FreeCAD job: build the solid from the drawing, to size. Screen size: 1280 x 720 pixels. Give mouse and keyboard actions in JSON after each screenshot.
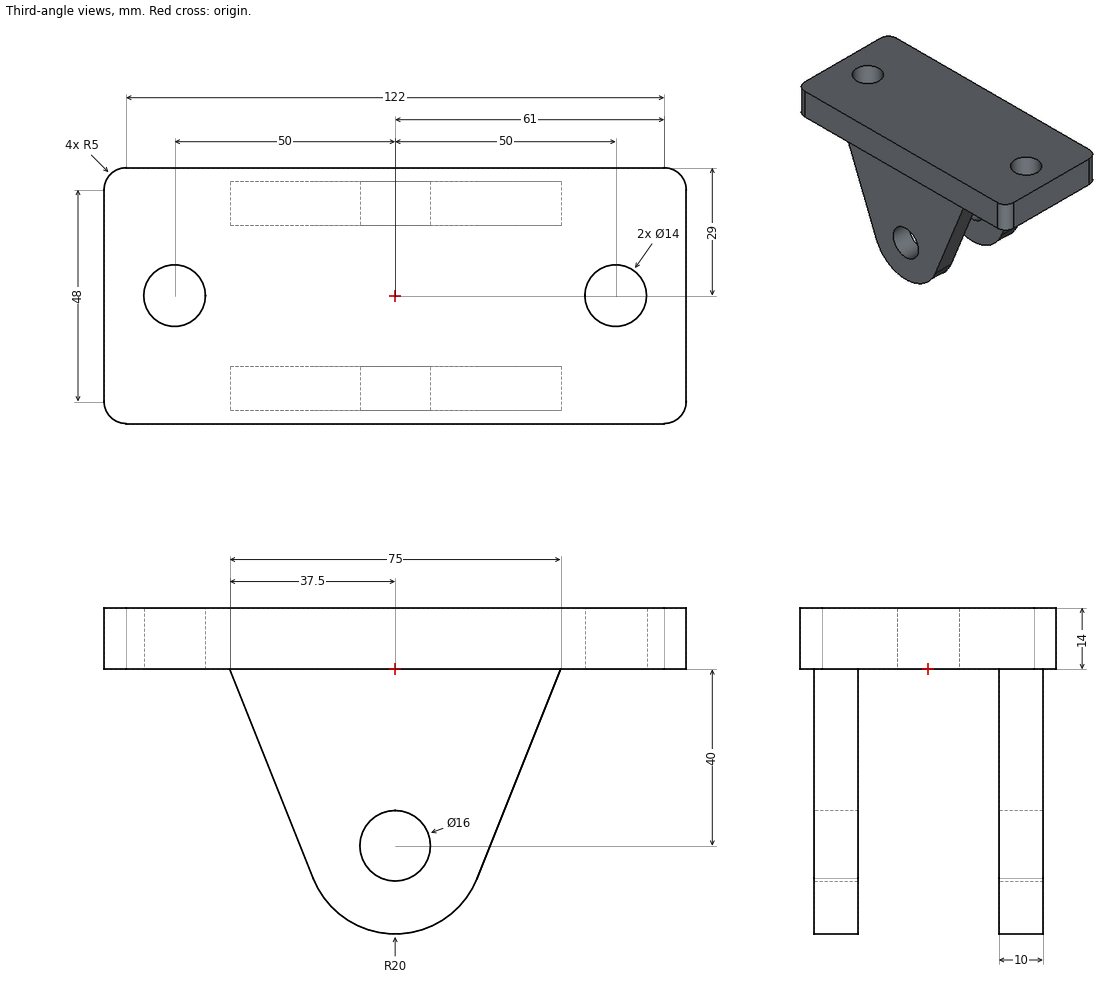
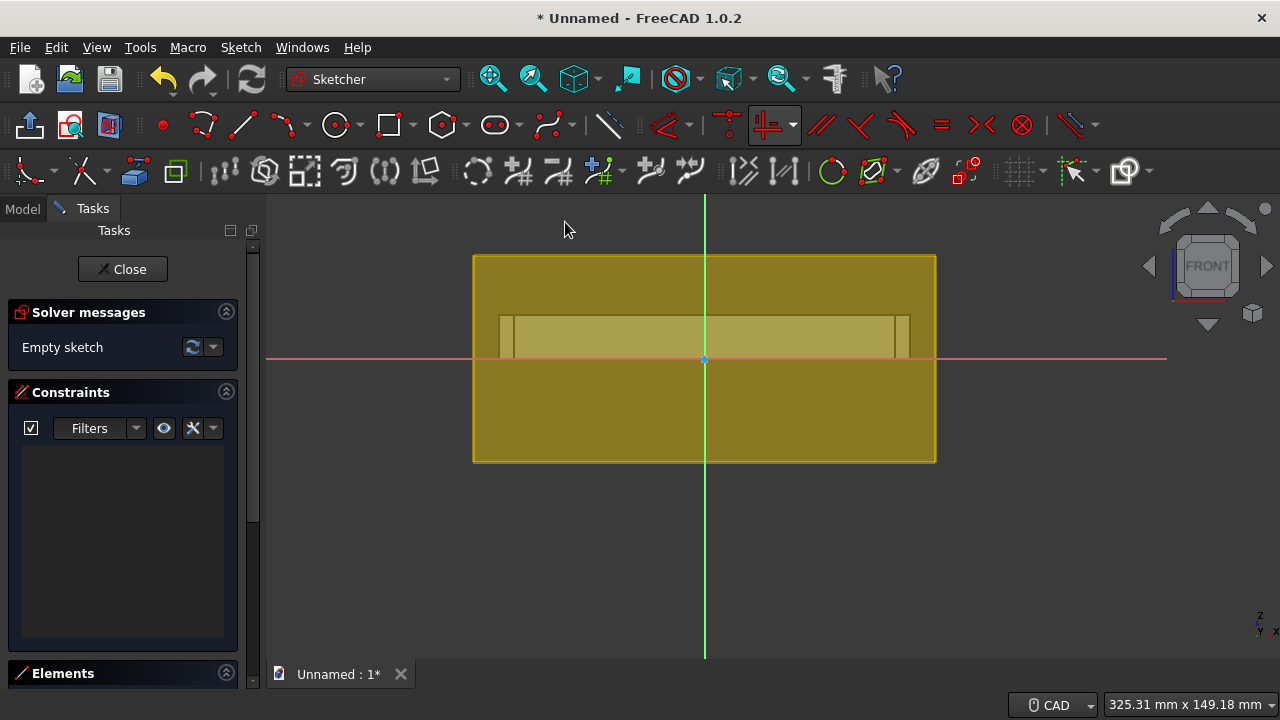
{"action": "scroll", "coordinate": [705, 506], "scroll_direction": "up", "scroll_amount": 2}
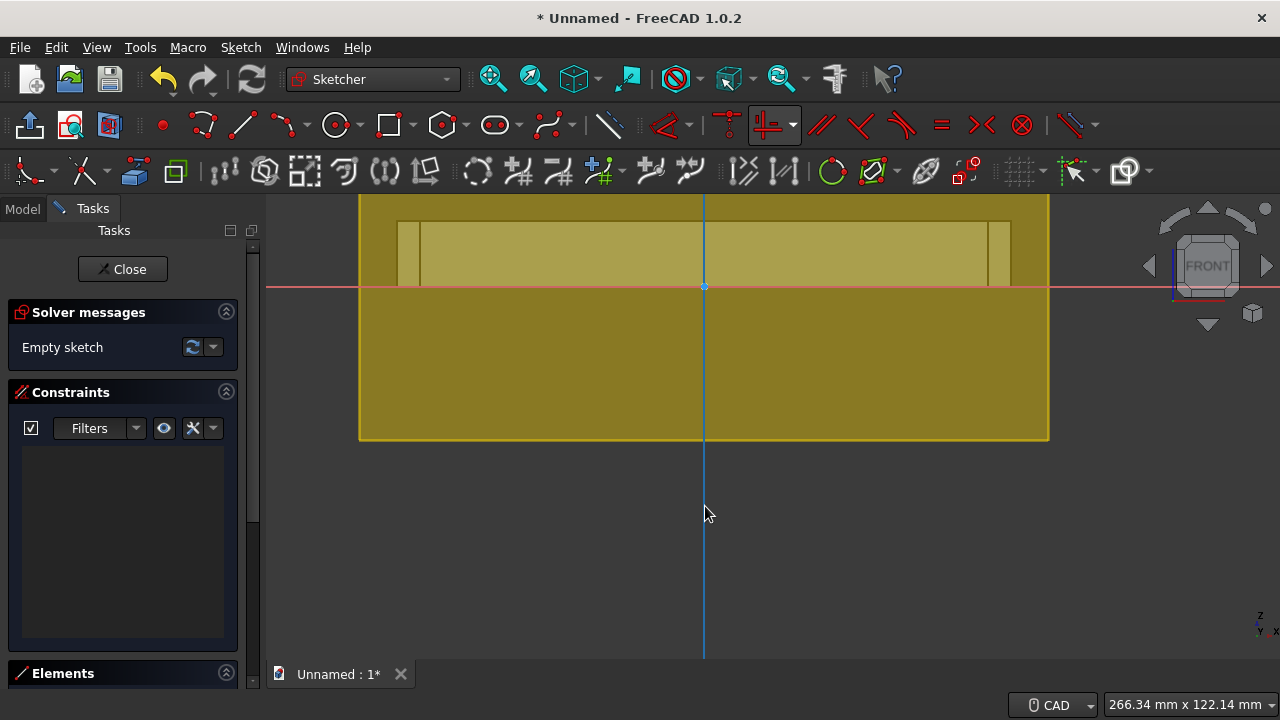
{"action": "left_click", "coordinate": [204, 126]}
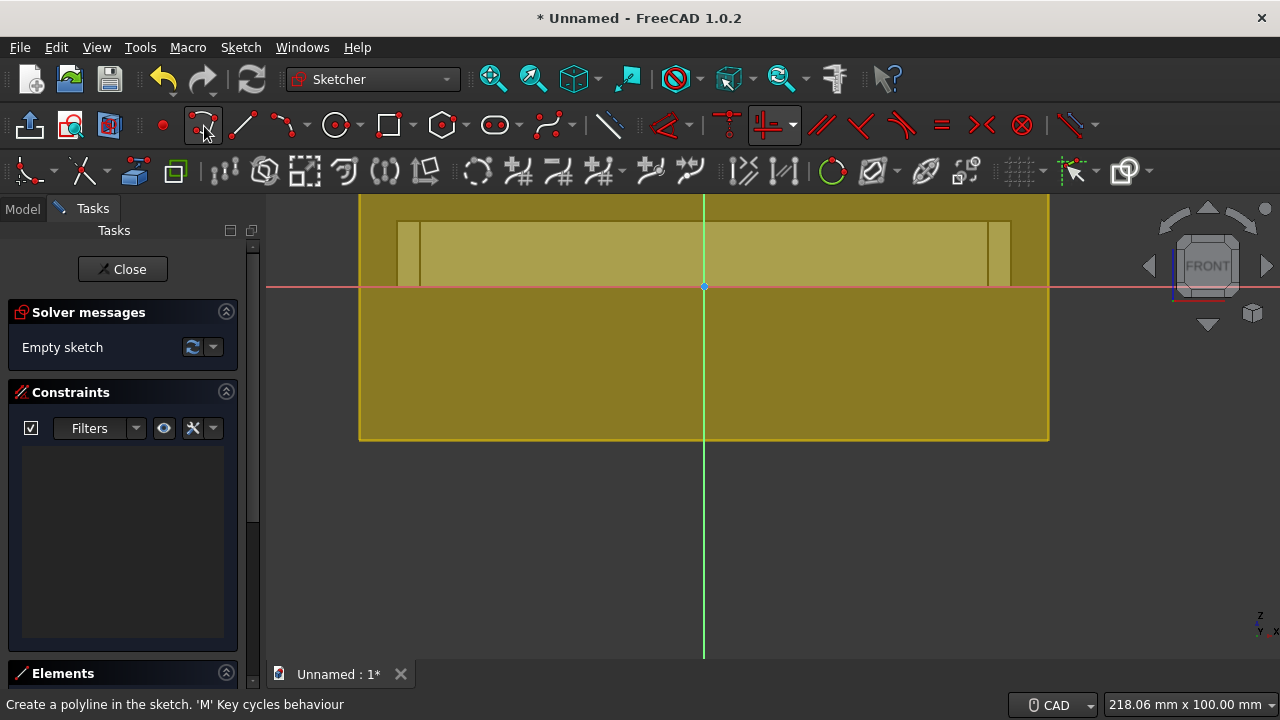
{"action": "left_click", "coordinate": [618, 507]}
{"action": "left_click", "coordinate": [530, 287]}
{"action": "left_click", "coordinate": [878, 296]}
{"action": "left_click", "coordinate": [790, 507]}
{"action": "right_click", "coordinate": [790, 507]}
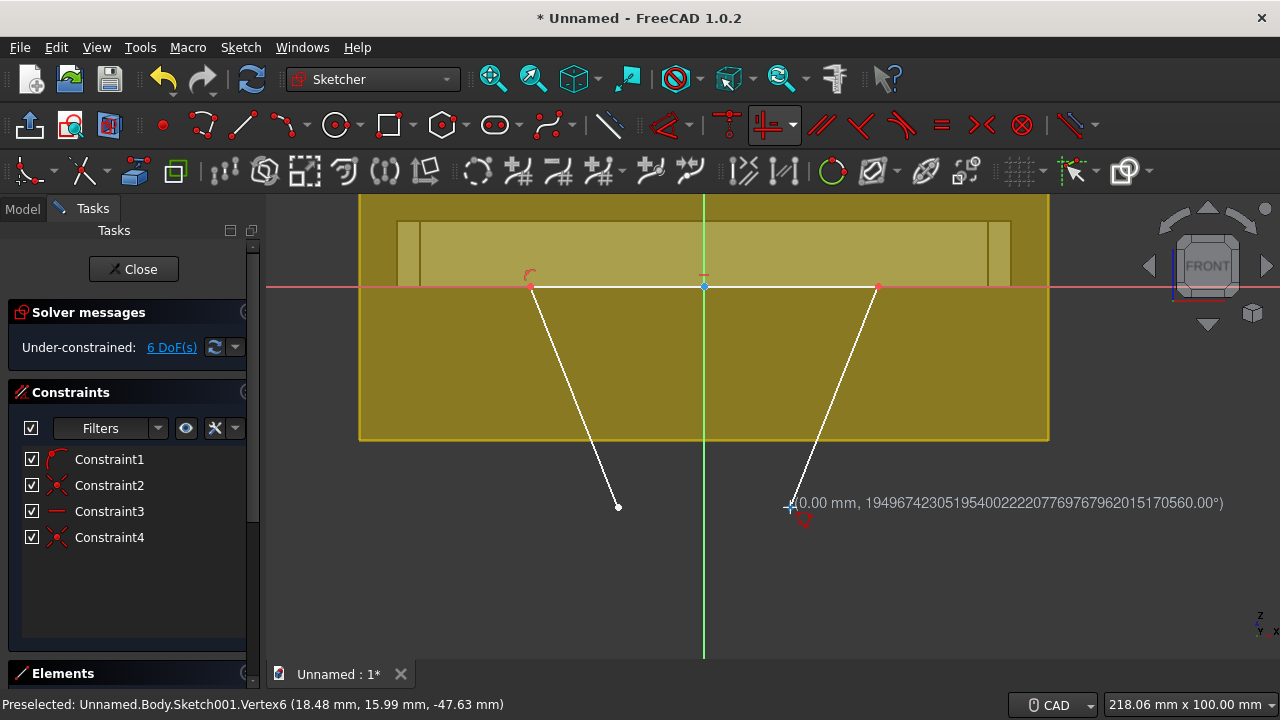
{"action": "left_click", "coordinate": [284, 126]}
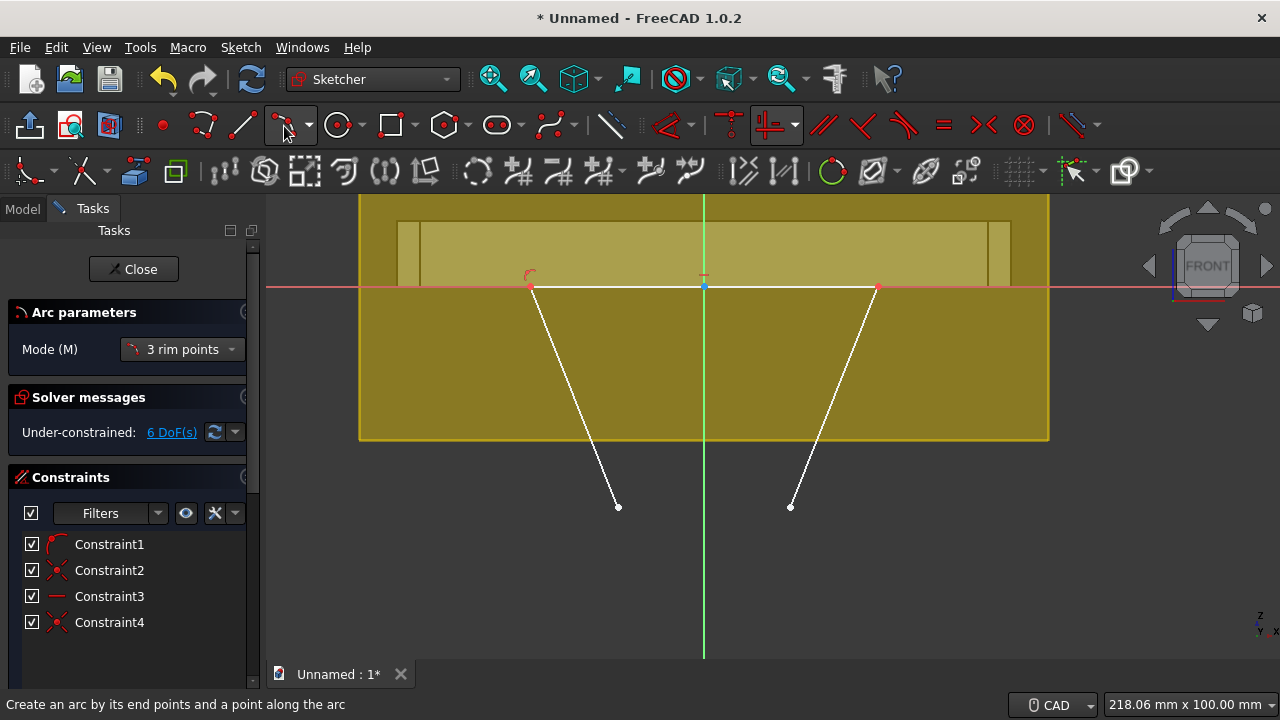
{"action": "left_click", "coordinate": [790, 508]}
{"action": "left_click", "coordinate": [618, 508]}
{"action": "left_click", "coordinate": [682, 563]}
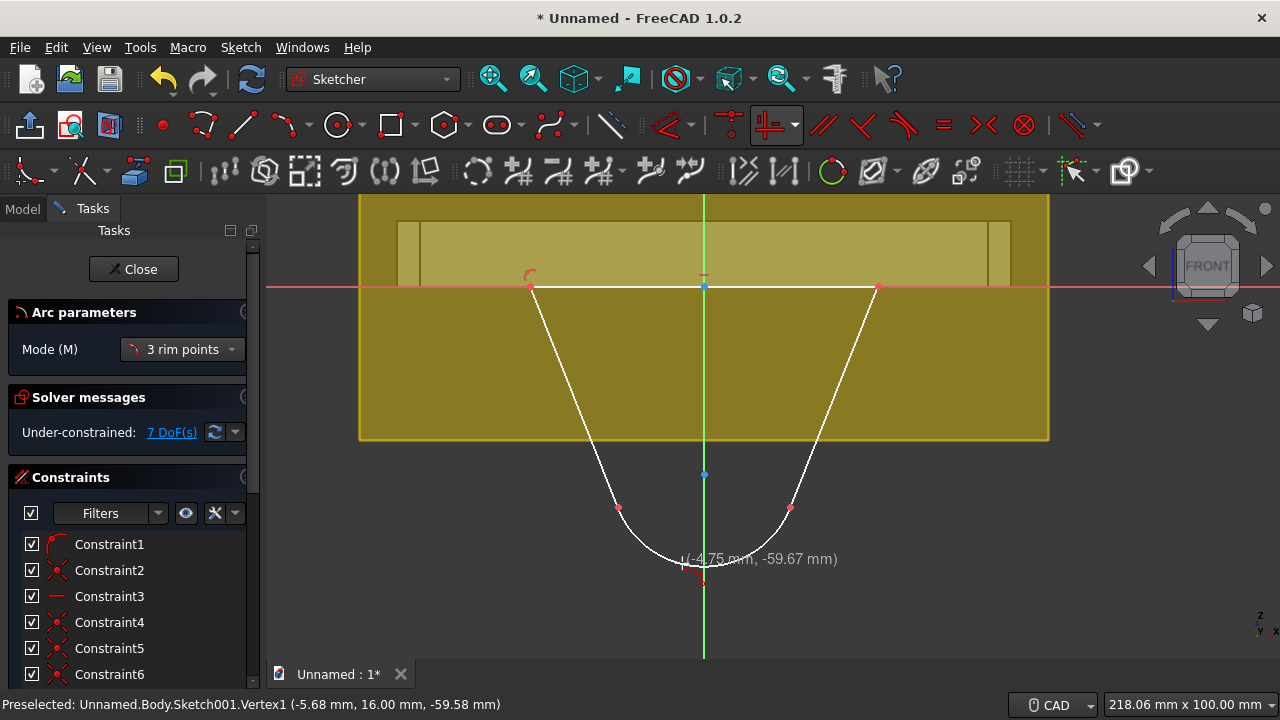
{"action": "left_click", "coordinate": [338, 126]}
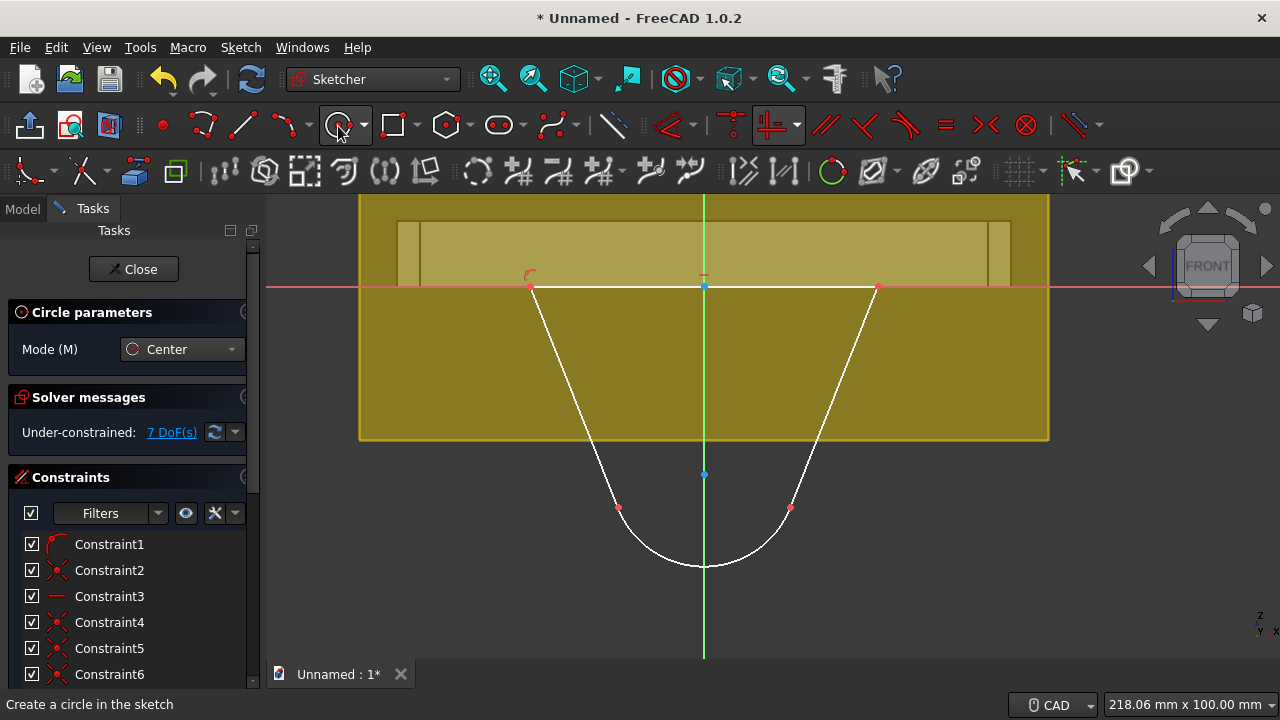
{"action": "left_click", "coordinate": [704, 473]}
{"action": "mouse_move", "coordinate": [730, 446]}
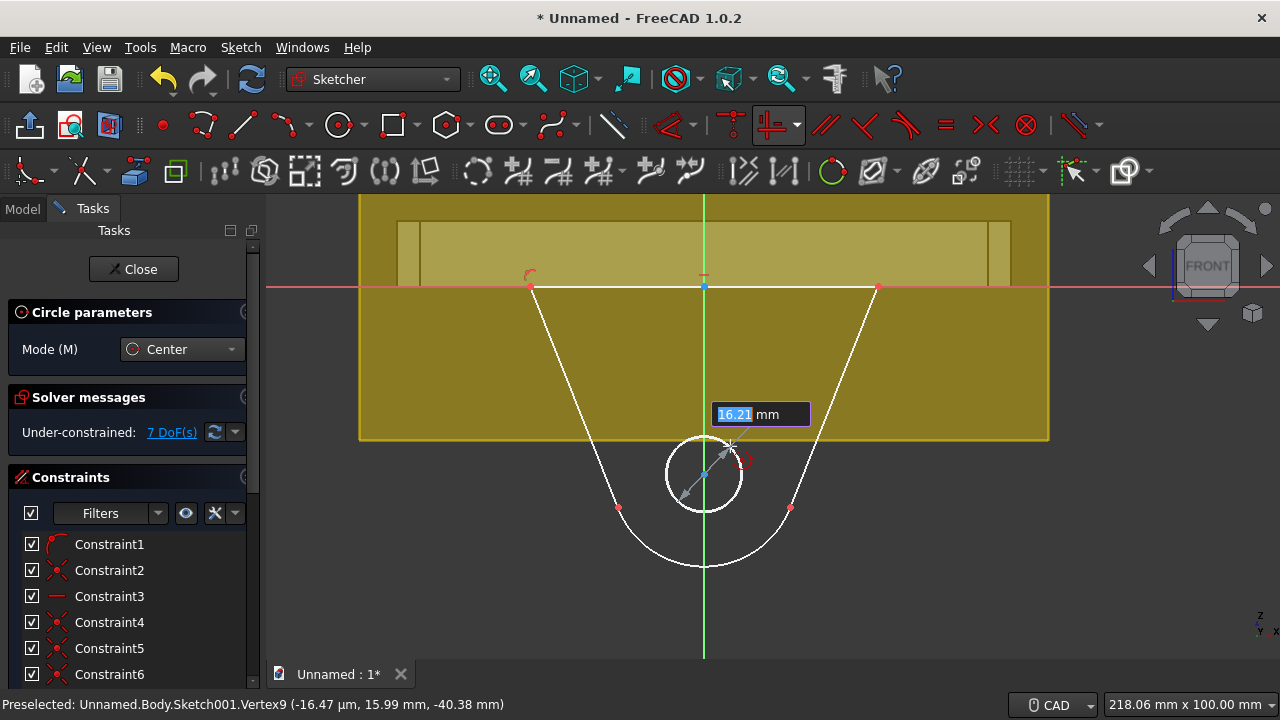
{"action": "type", "text": "16"}
{"action": "key", "text": "Return"}
{"action": "key", "text": "Escape"}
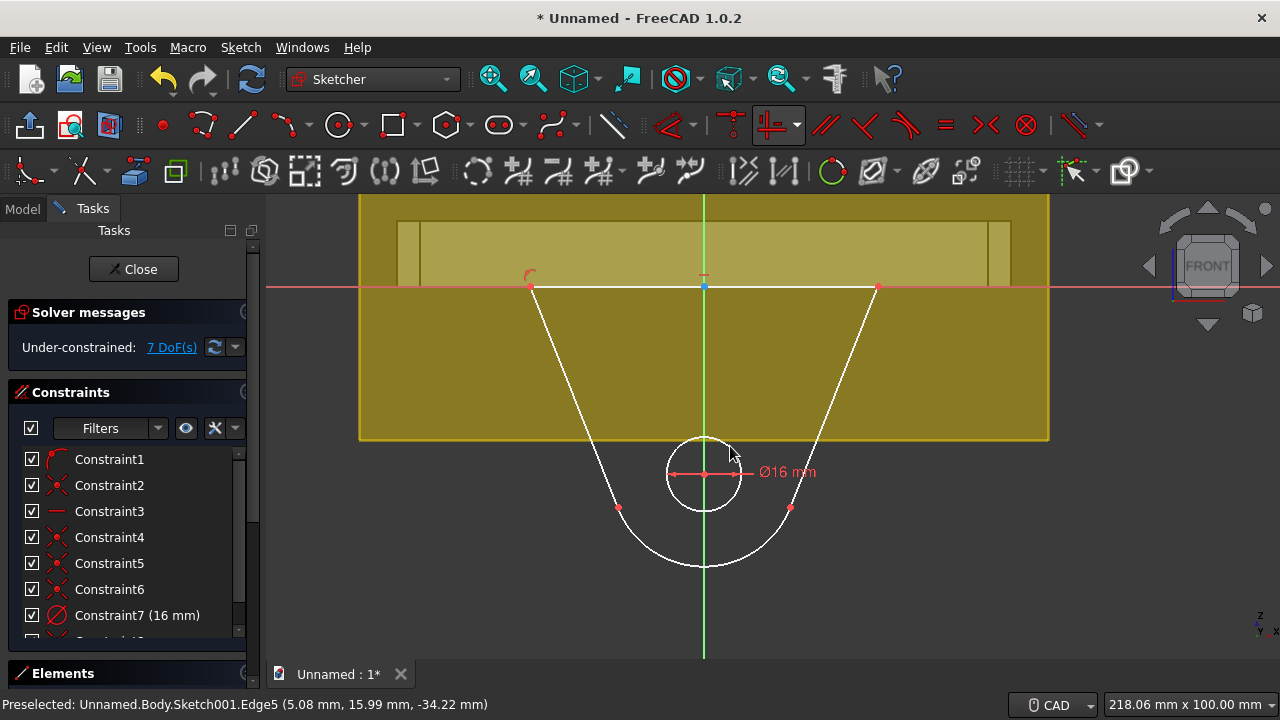
{"action": "left_click", "coordinate": [592, 442]}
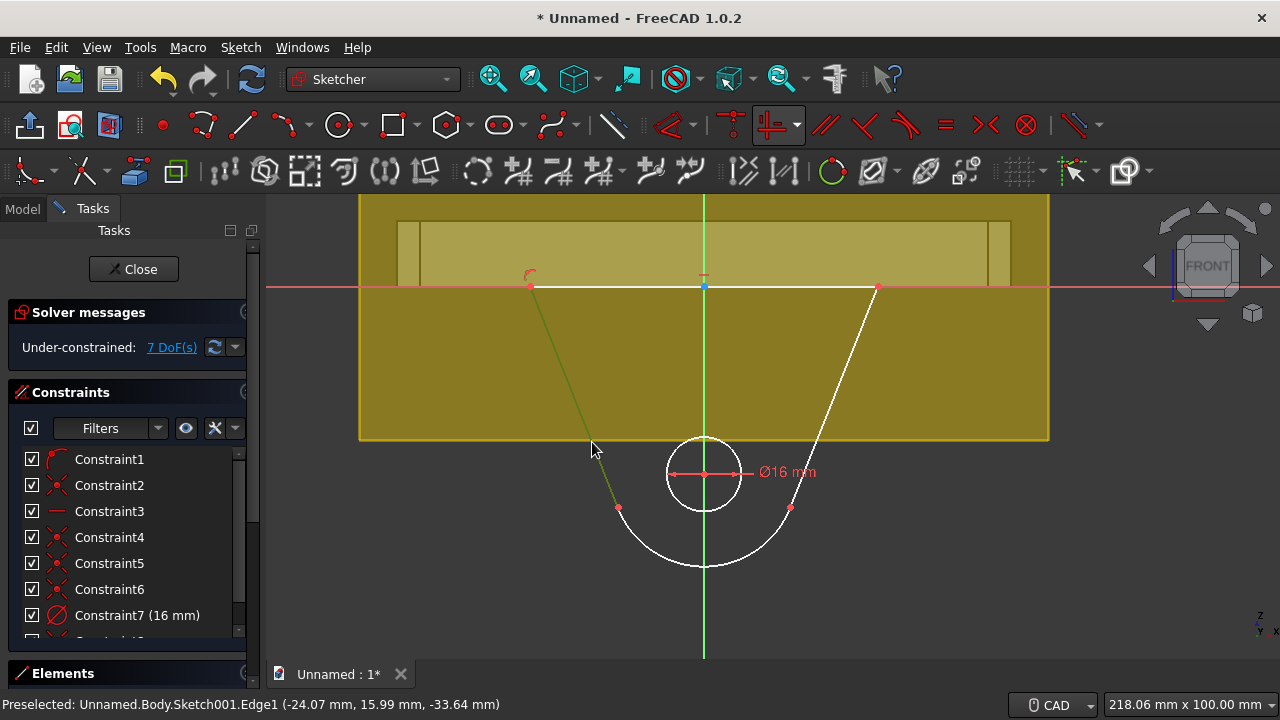
{"action": "left_click", "coordinate": [661, 556]}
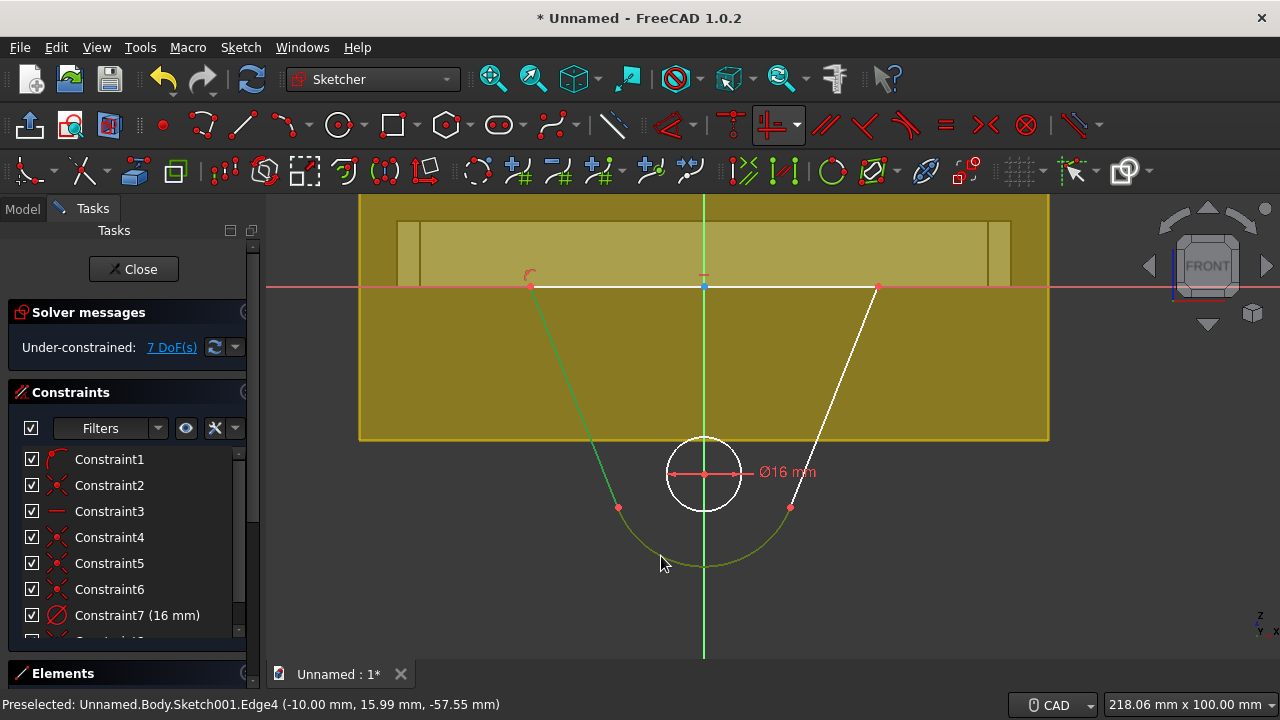
{"action": "left_click", "coordinate": [906, 126]}